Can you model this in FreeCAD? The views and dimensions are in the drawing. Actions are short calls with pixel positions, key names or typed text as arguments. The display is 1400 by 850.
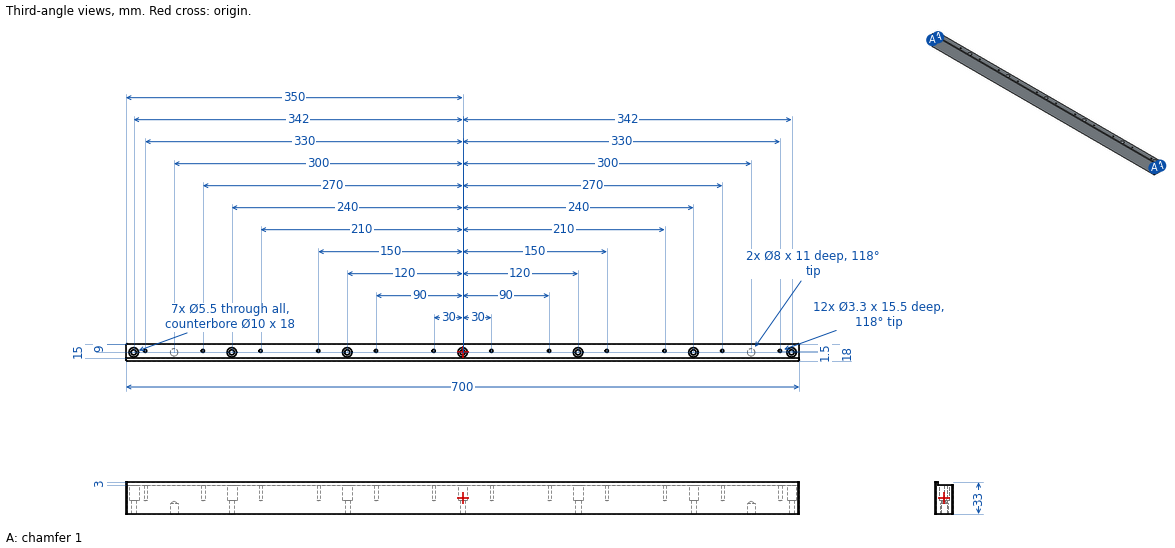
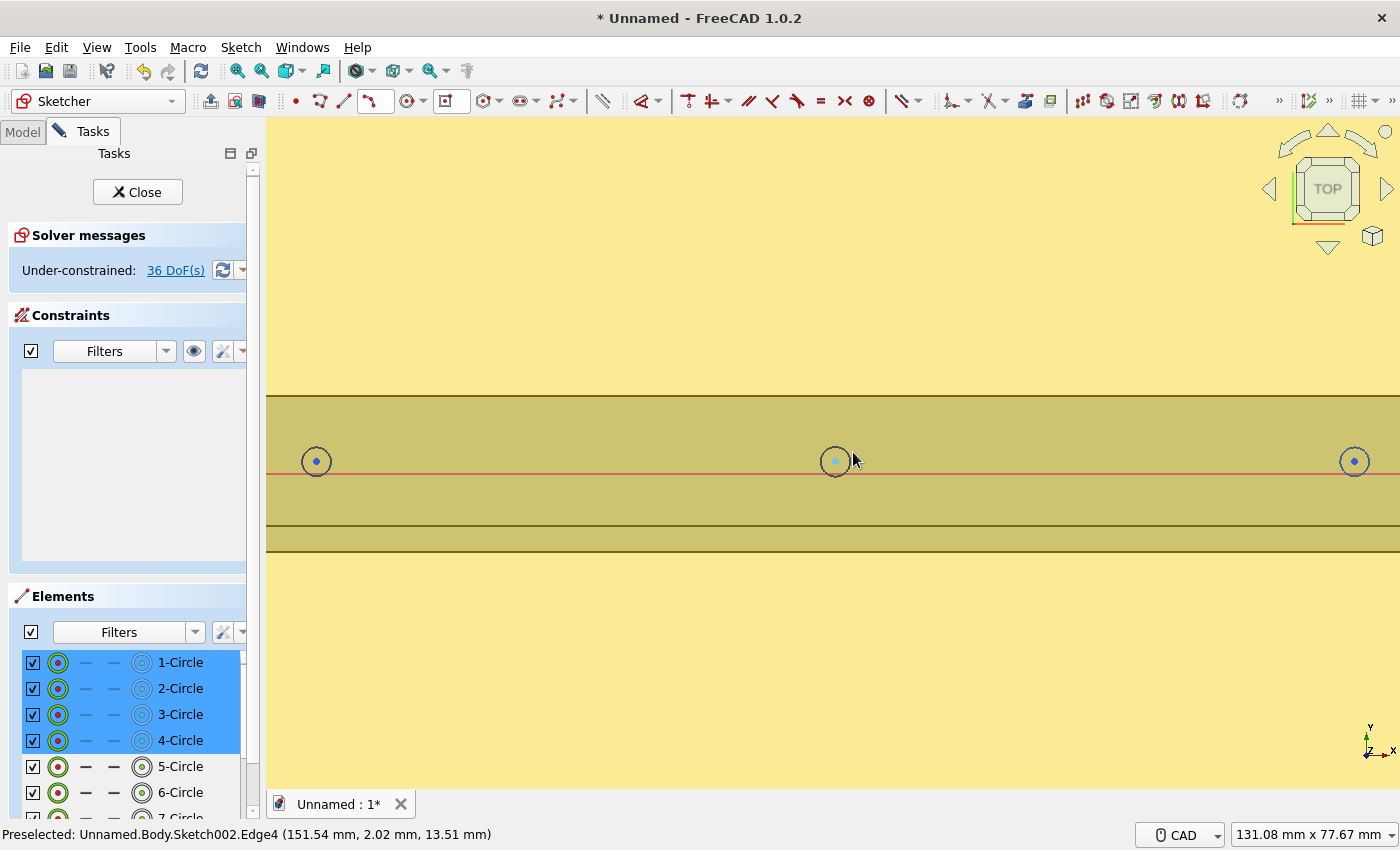
click(846, 451)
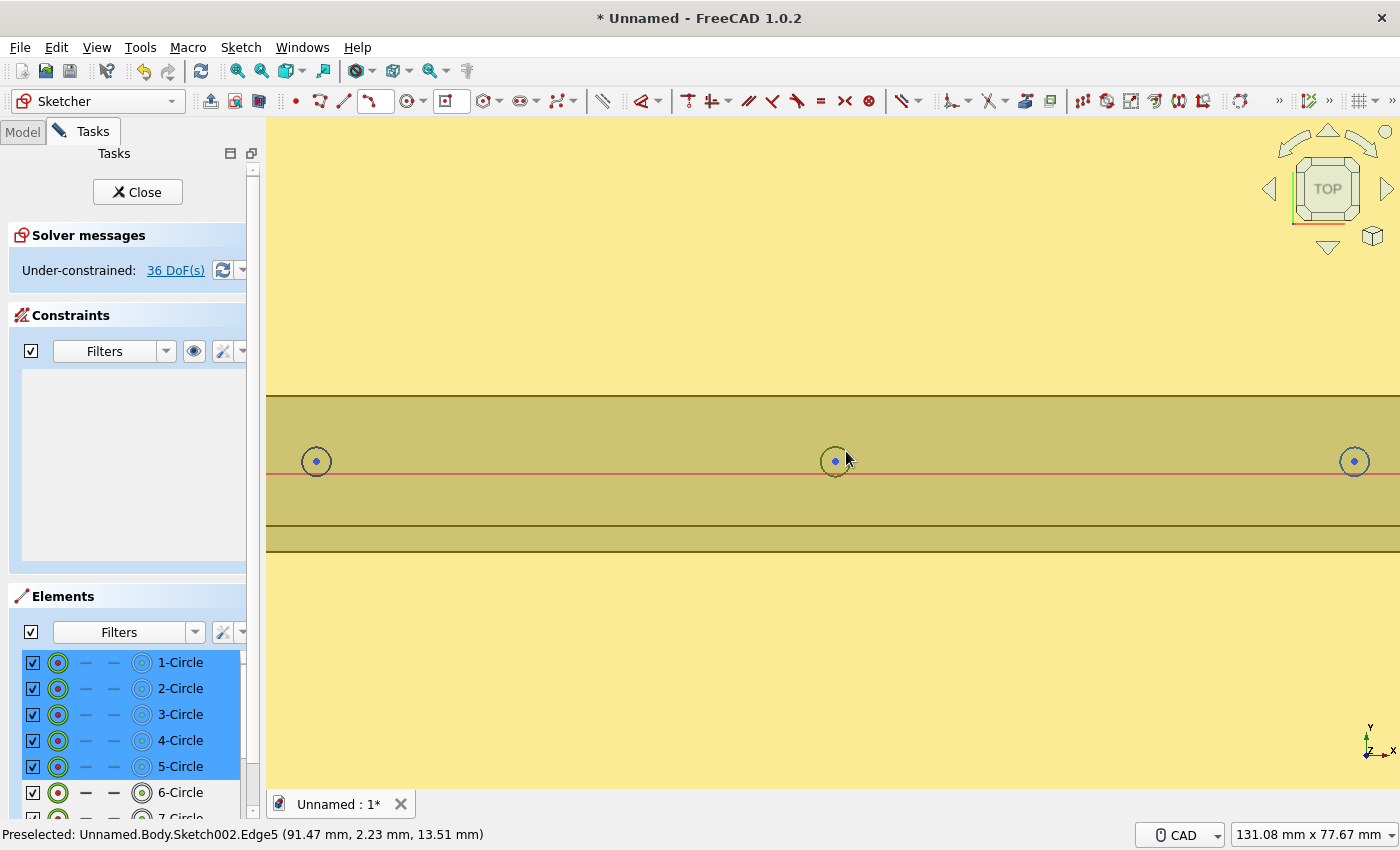
click(327, 452)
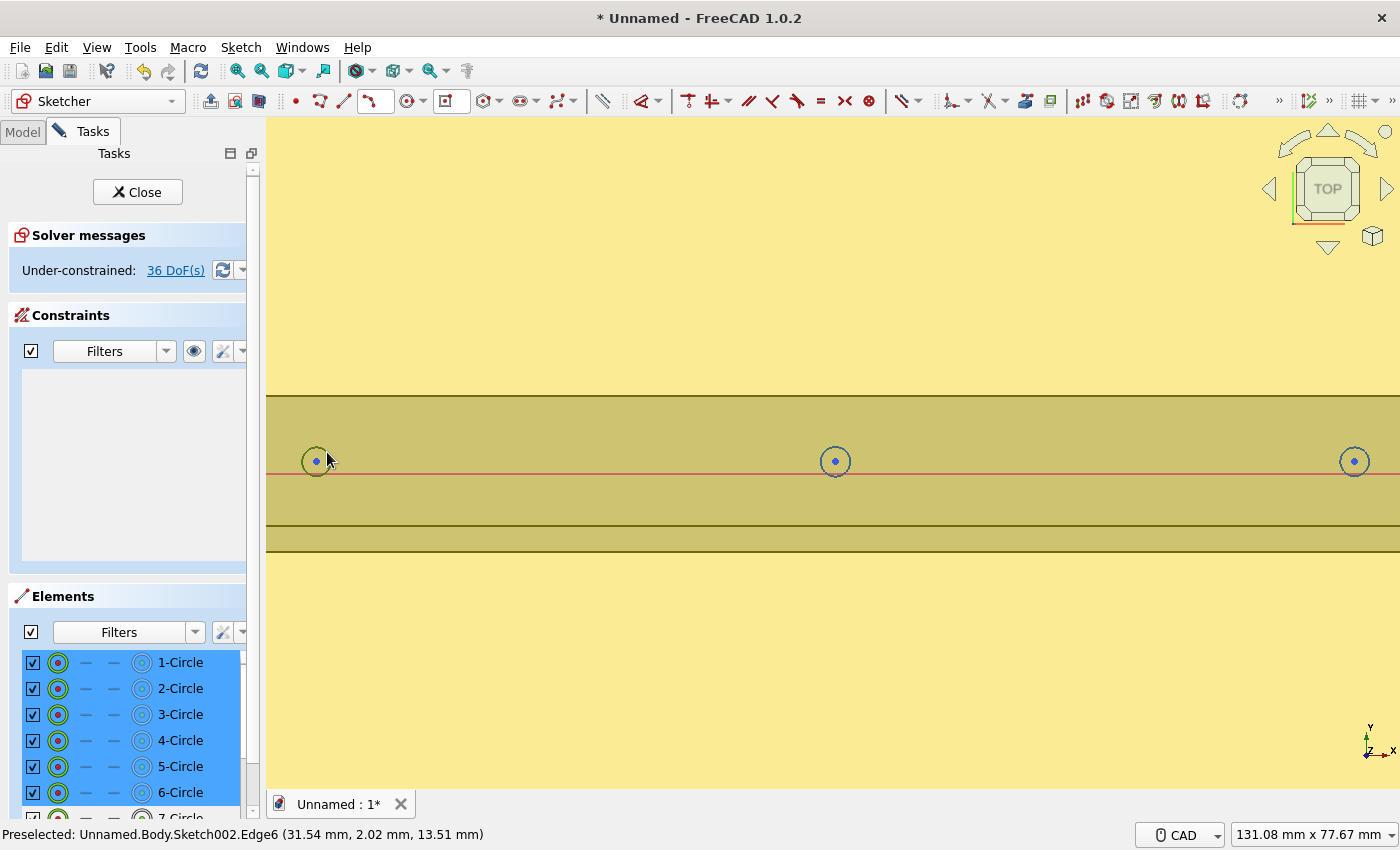
scroll(853, 452, down, 11)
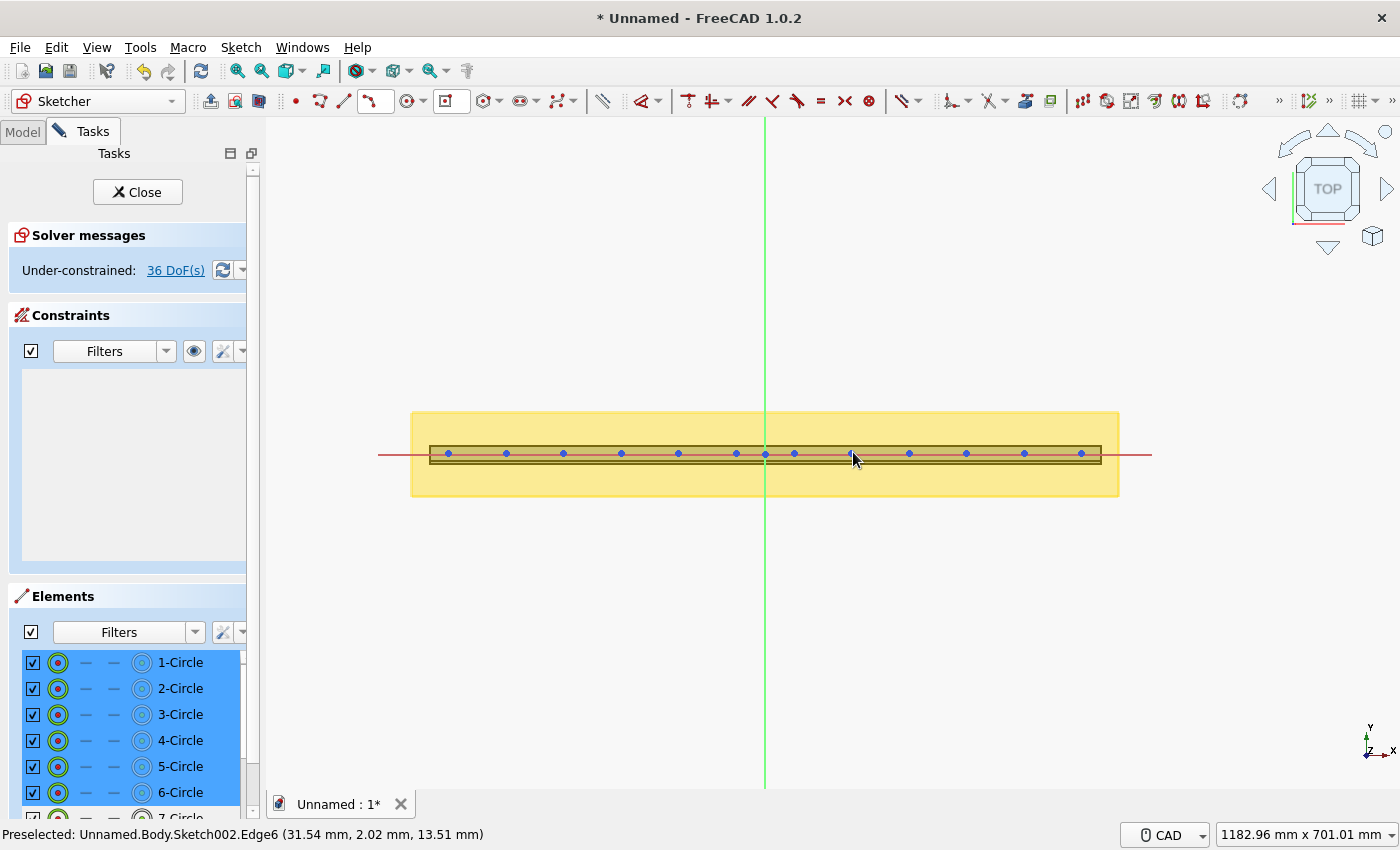
scroll(738, 452, up, 11)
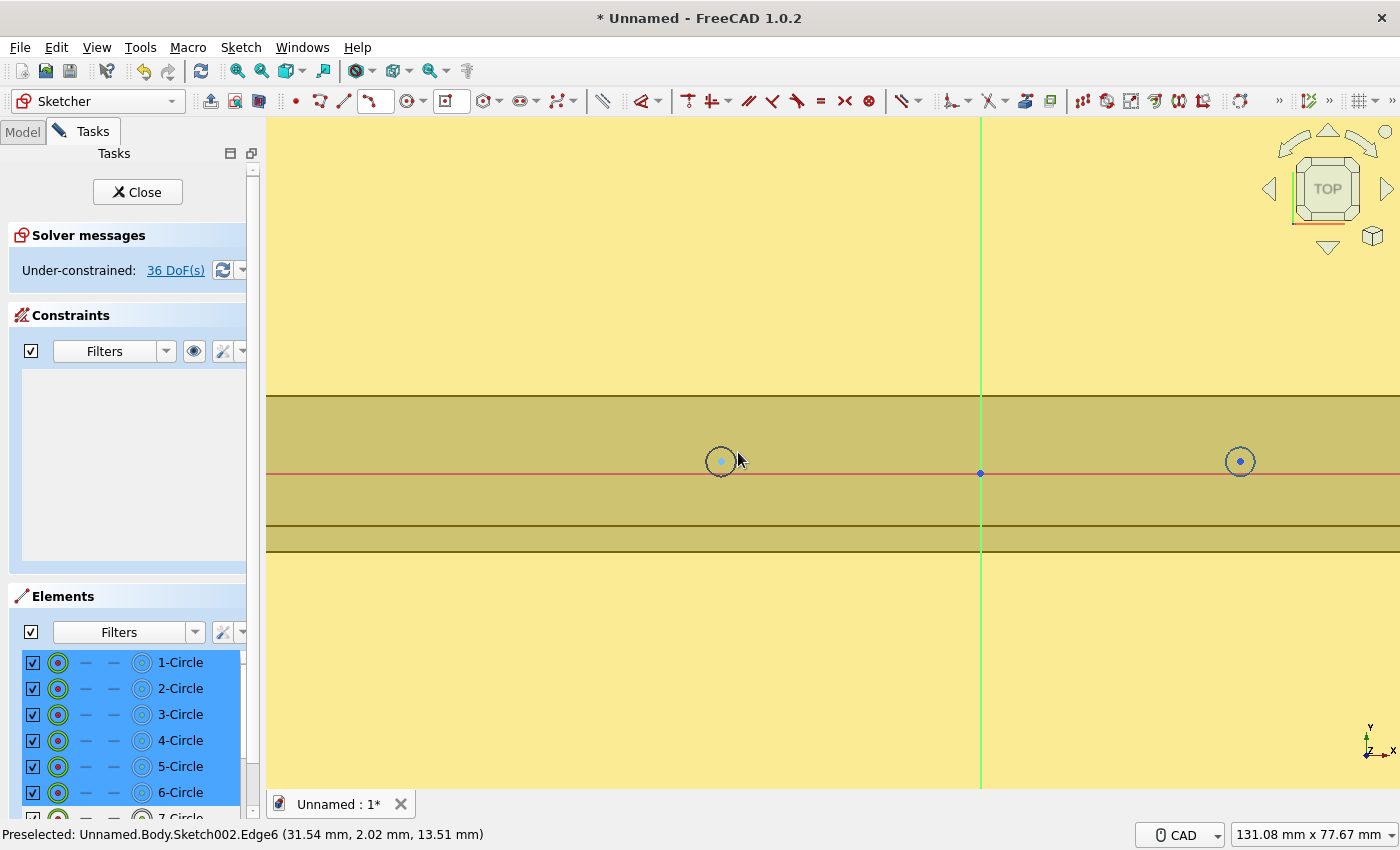
click(731, 451)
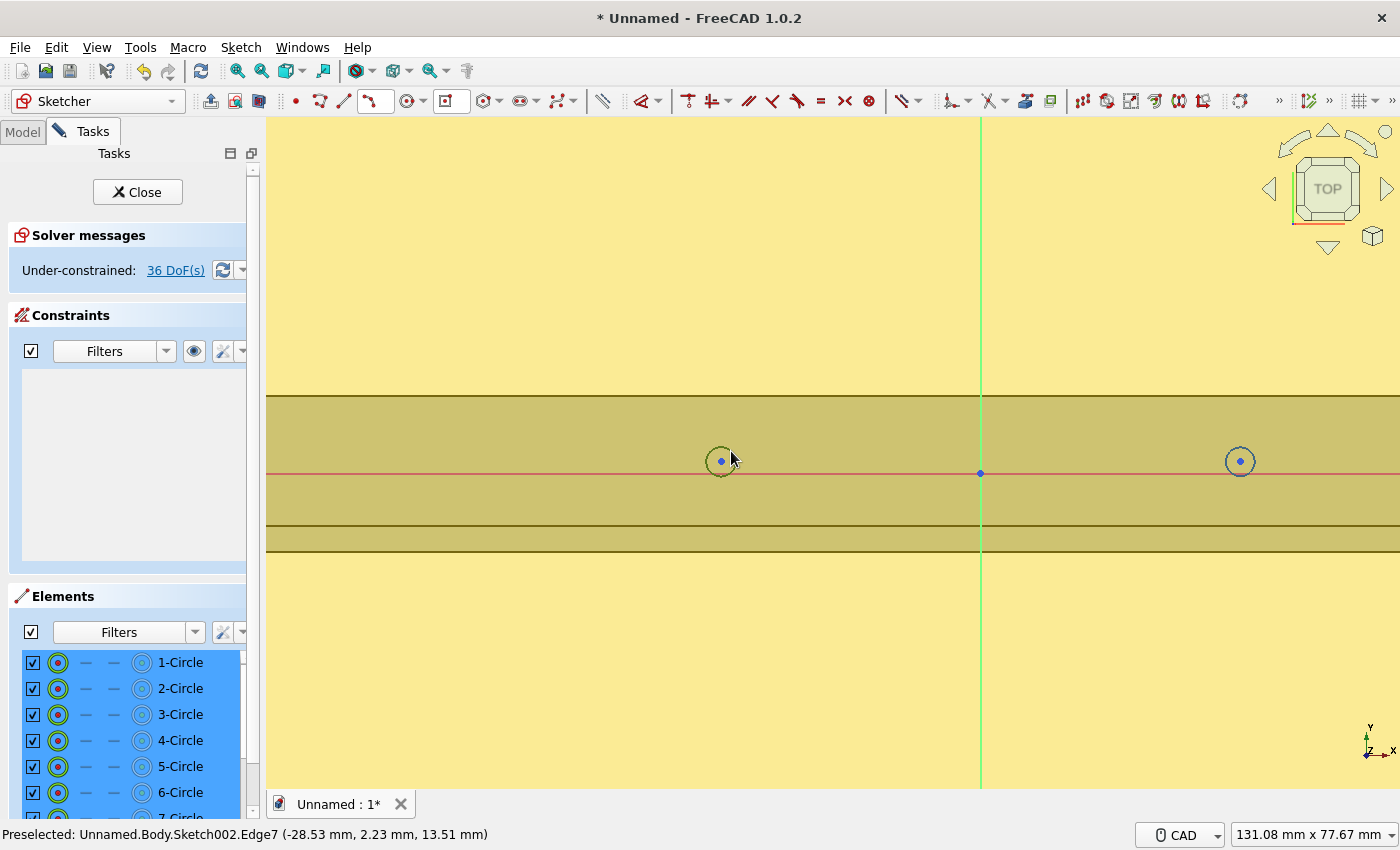
scroll(738, 452, down, 11)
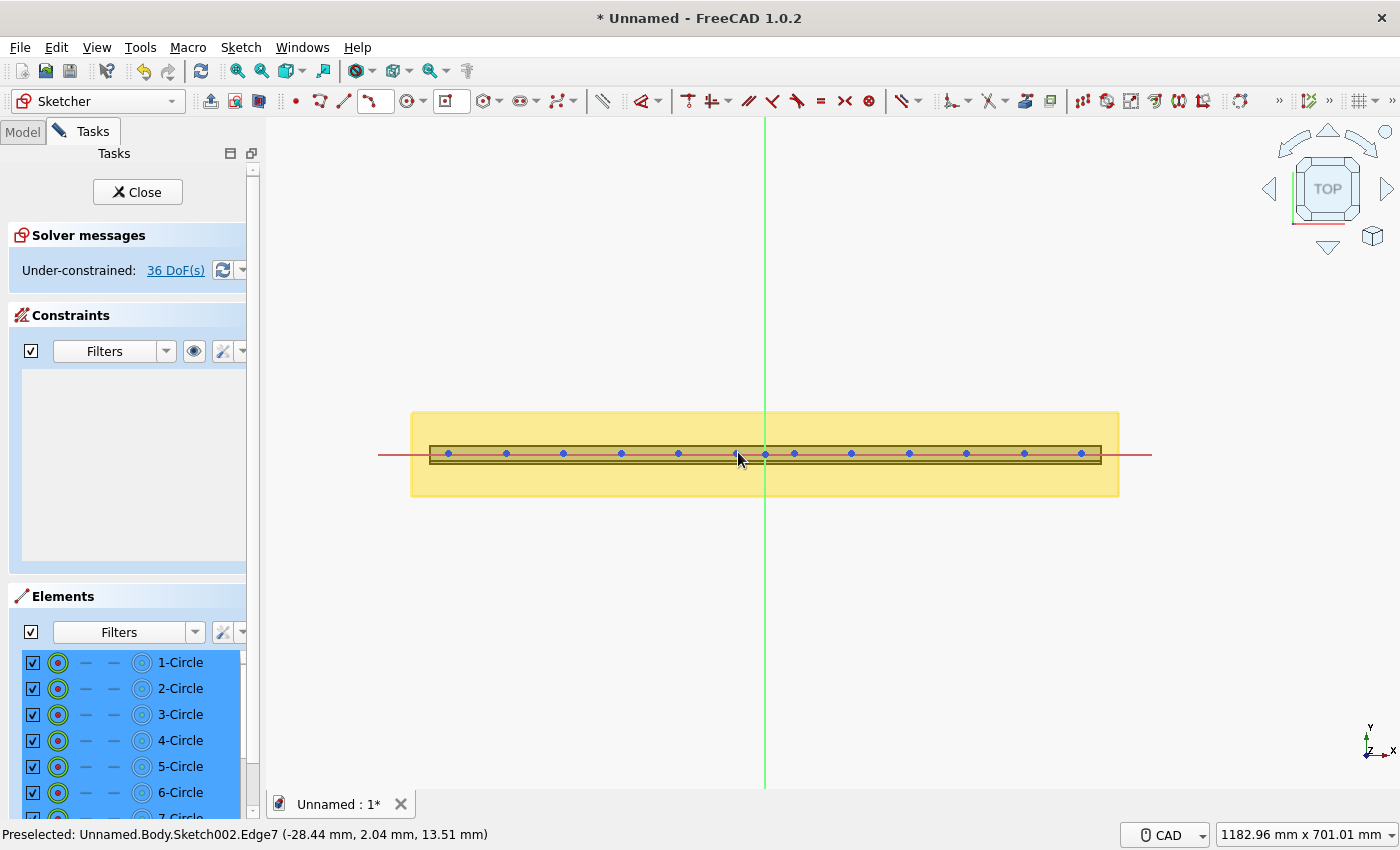
scroll(680, 452, up, 11)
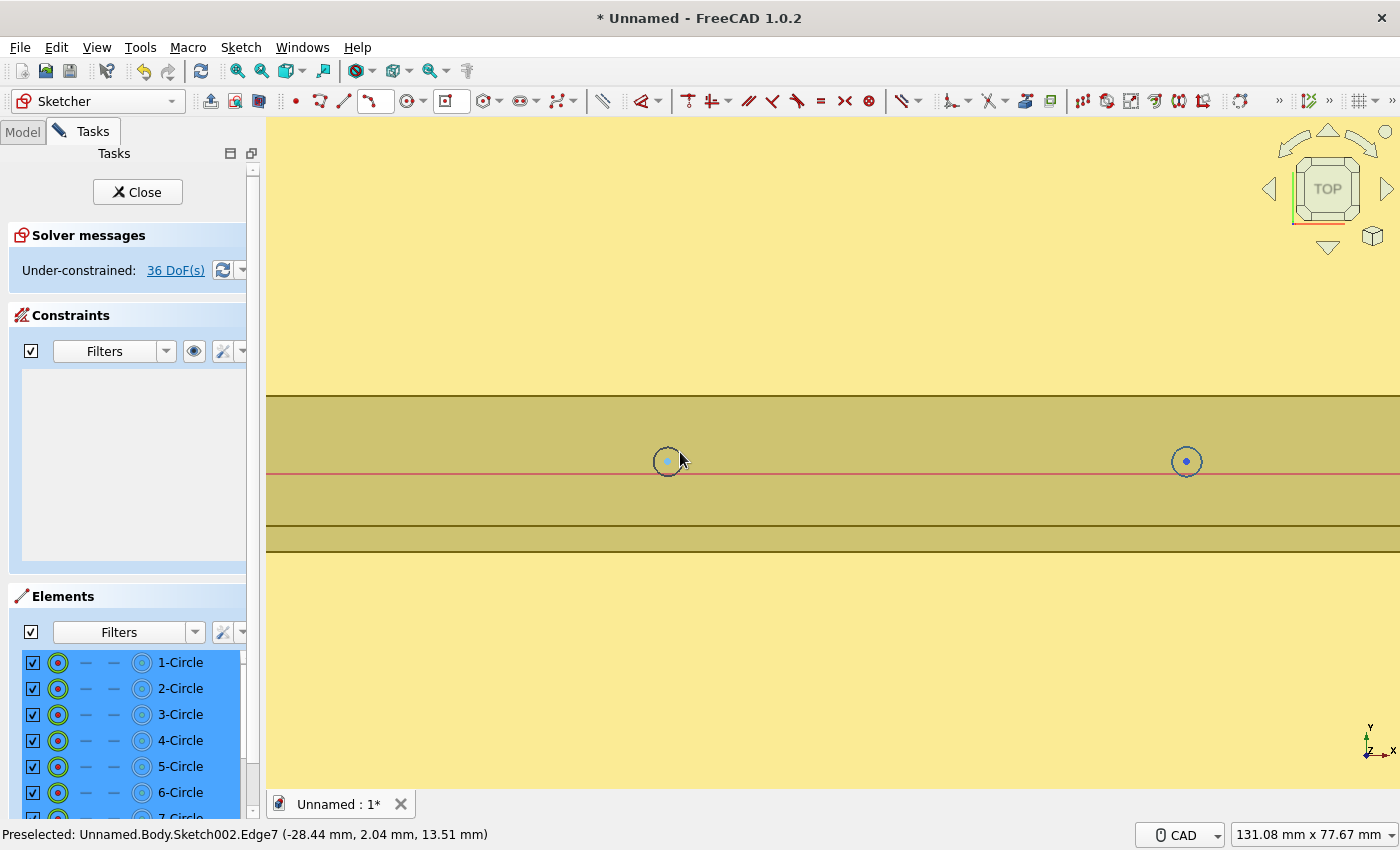
click(678, 452)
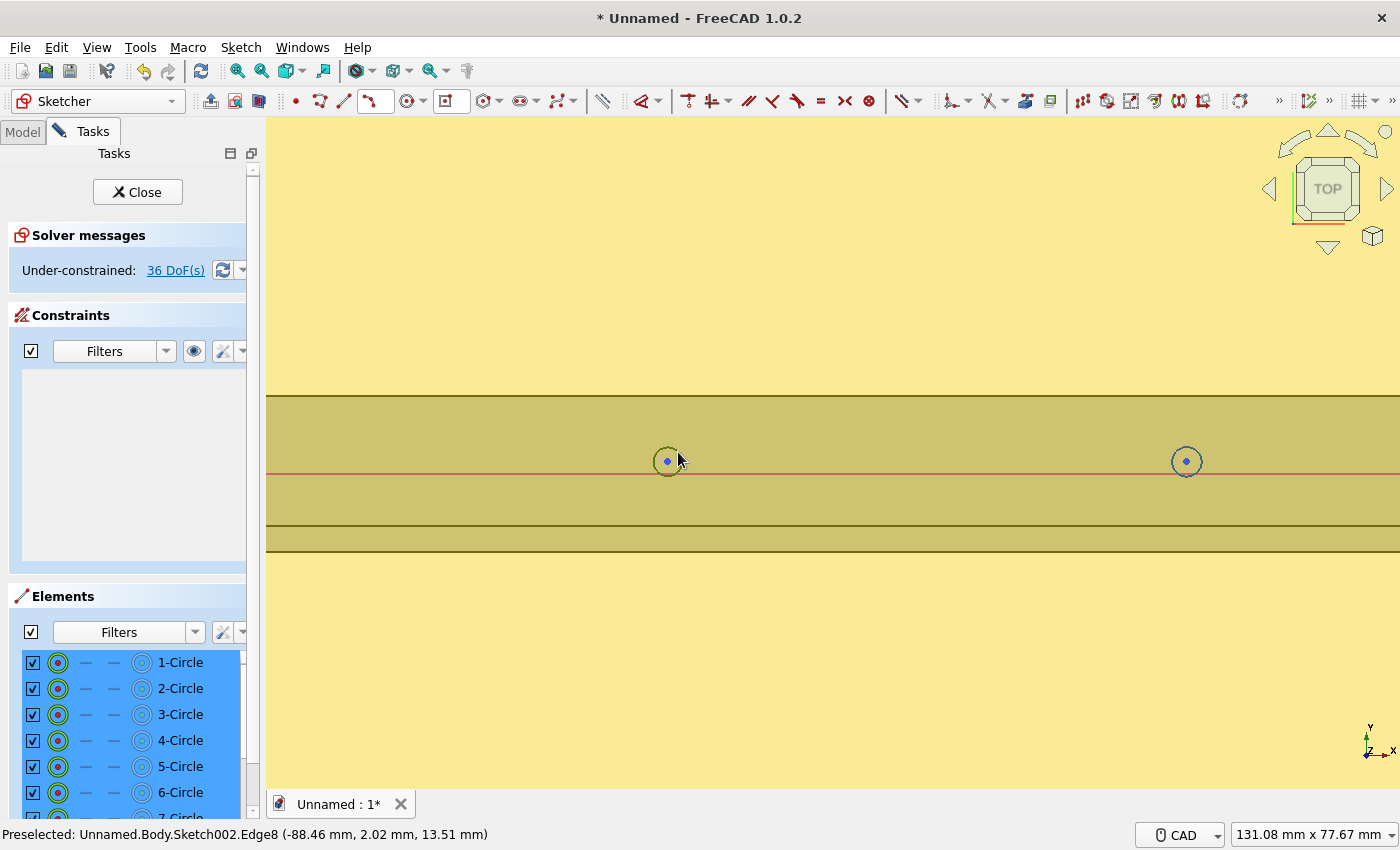
scroll(680, 452, down, 11)